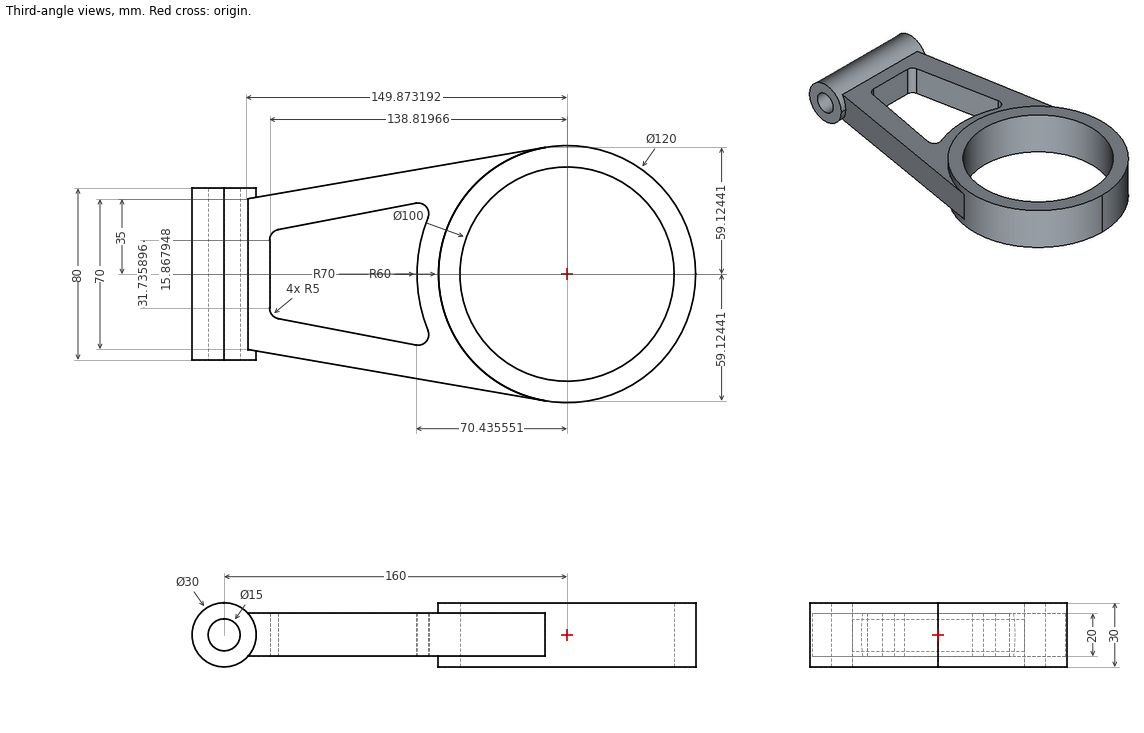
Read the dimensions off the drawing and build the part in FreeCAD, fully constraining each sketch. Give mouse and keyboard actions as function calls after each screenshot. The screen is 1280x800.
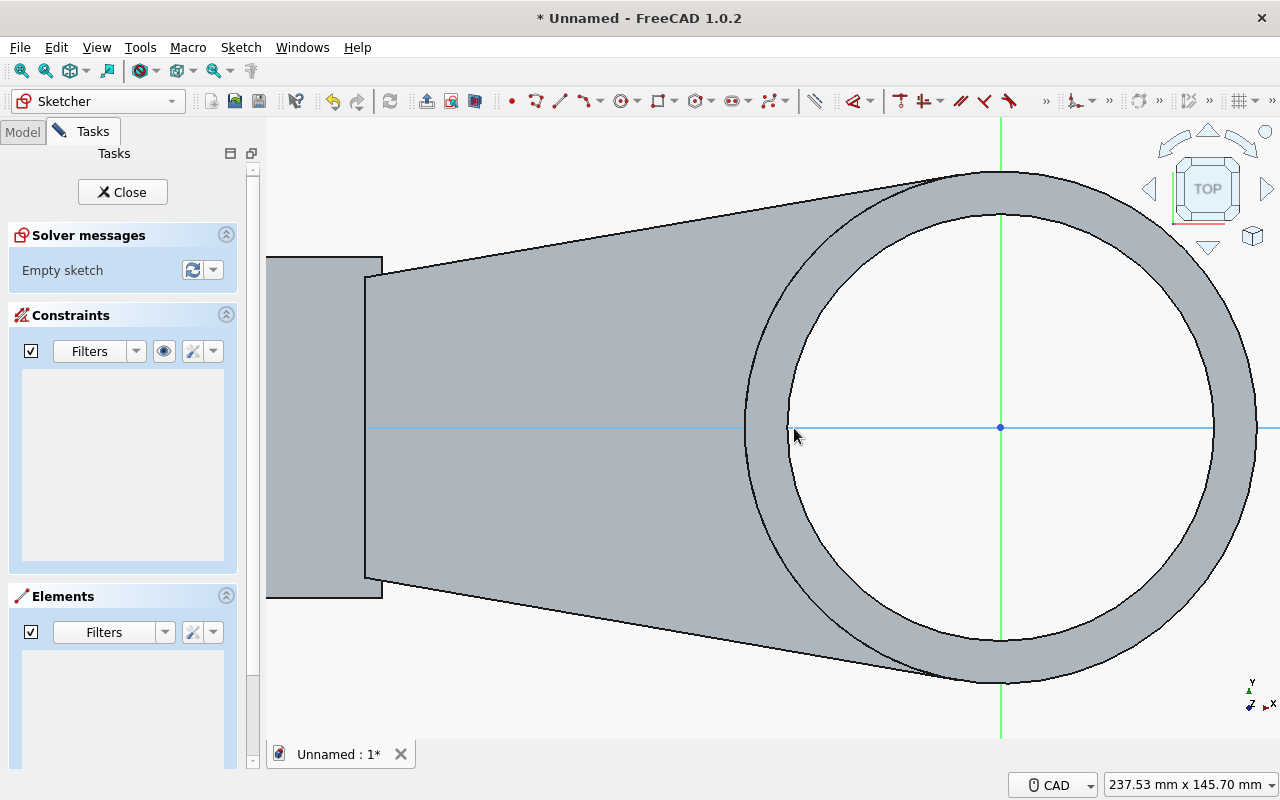
click(560, 102)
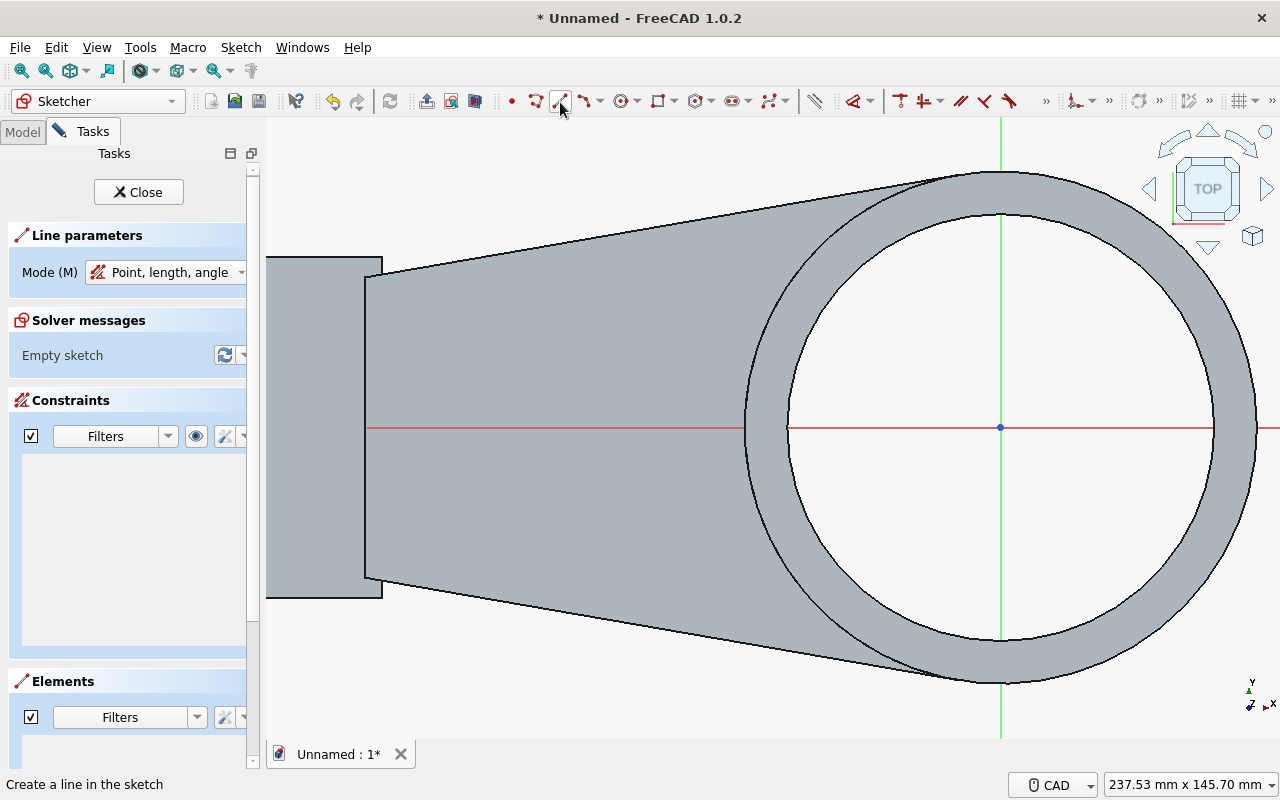
click(408, 360)
click(408, 495)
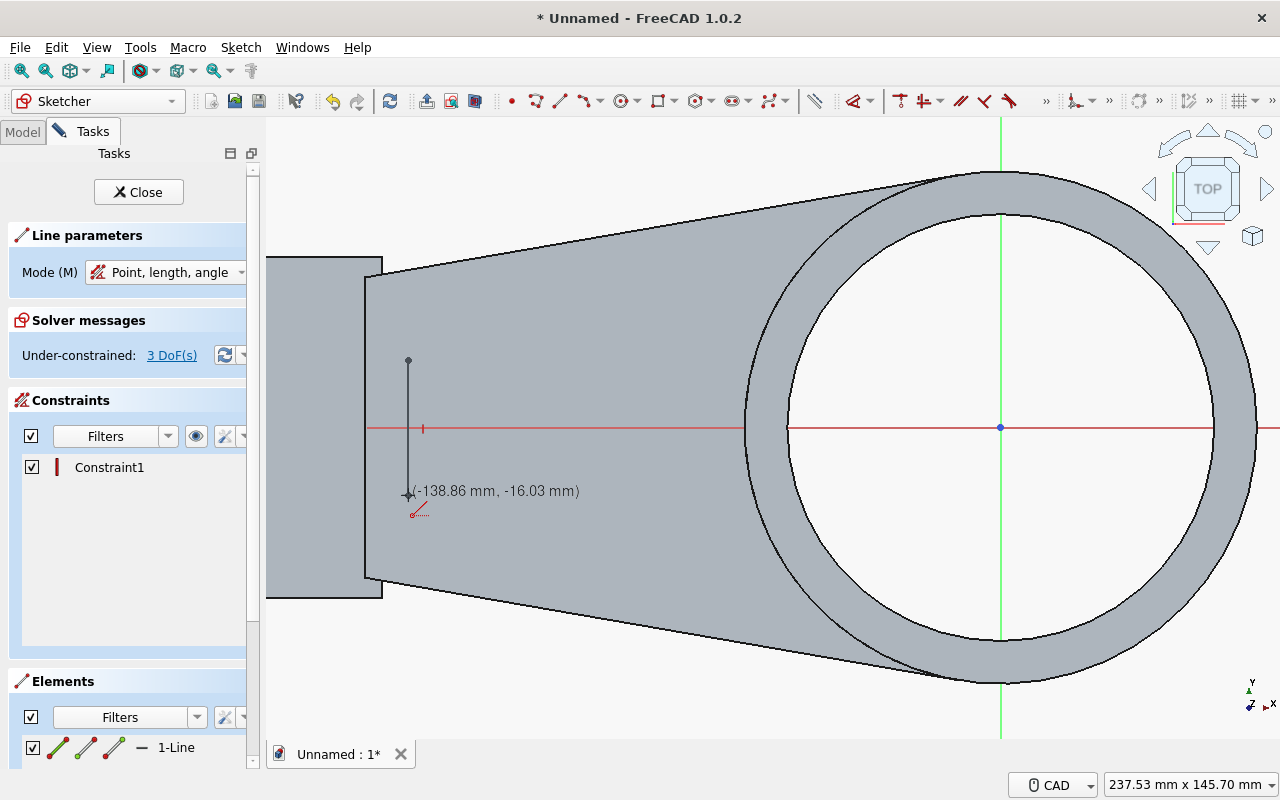
click(425, 516)
click(700, 569)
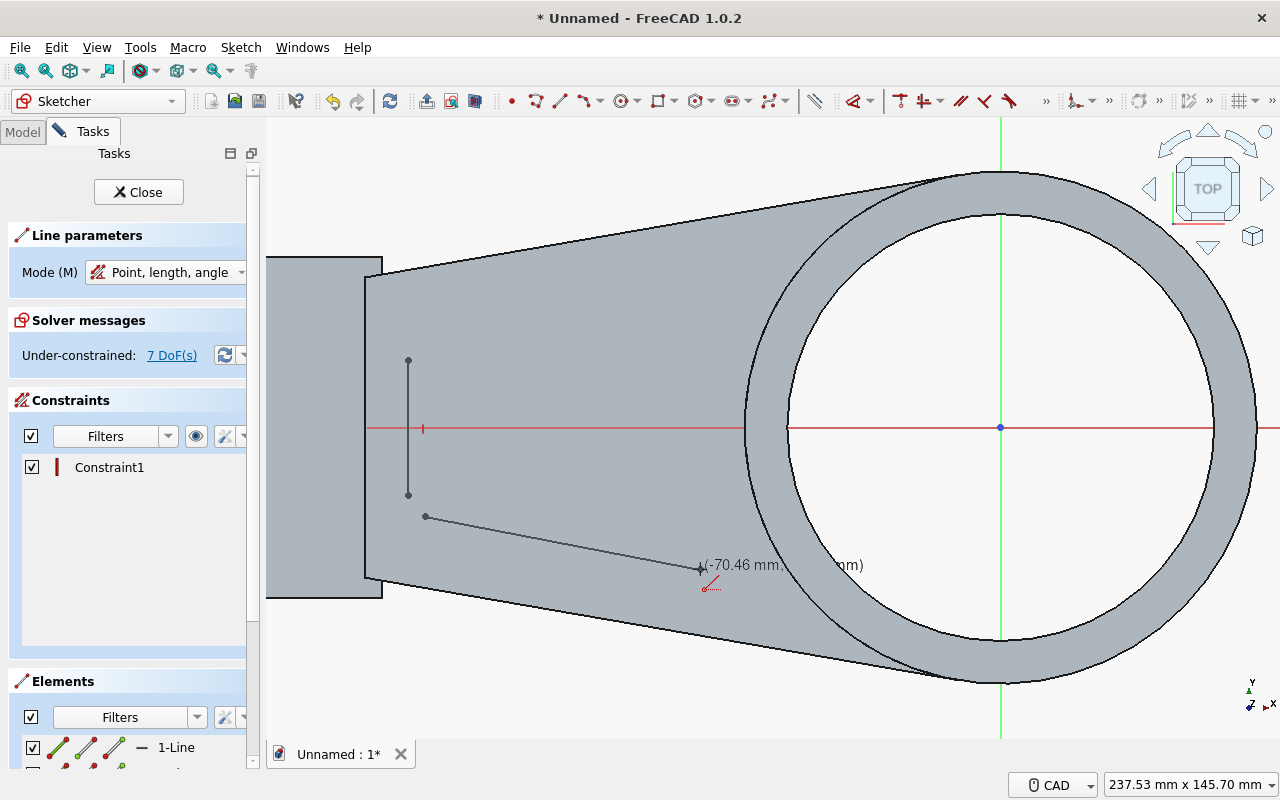
click(700, 286)
click(425, 339)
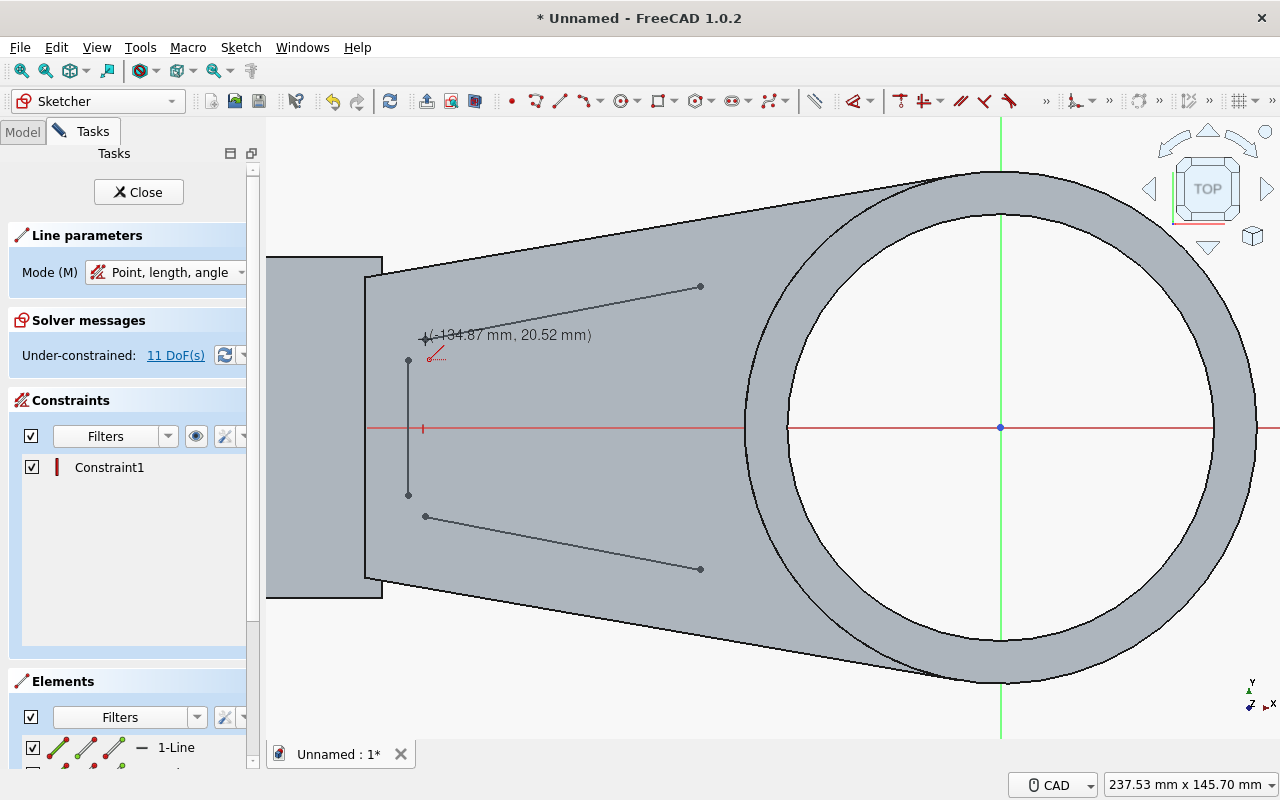
click(584, 102)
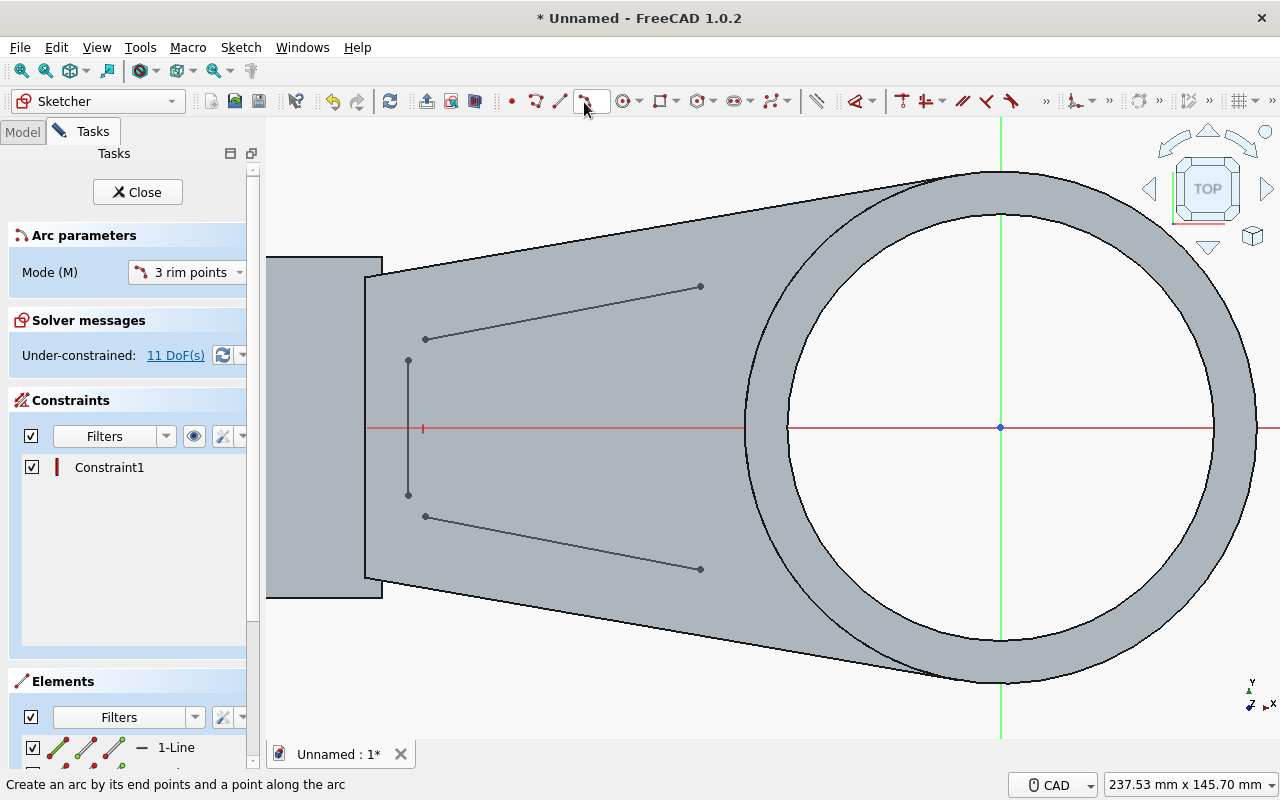
click(408, 496)
click(425, 517)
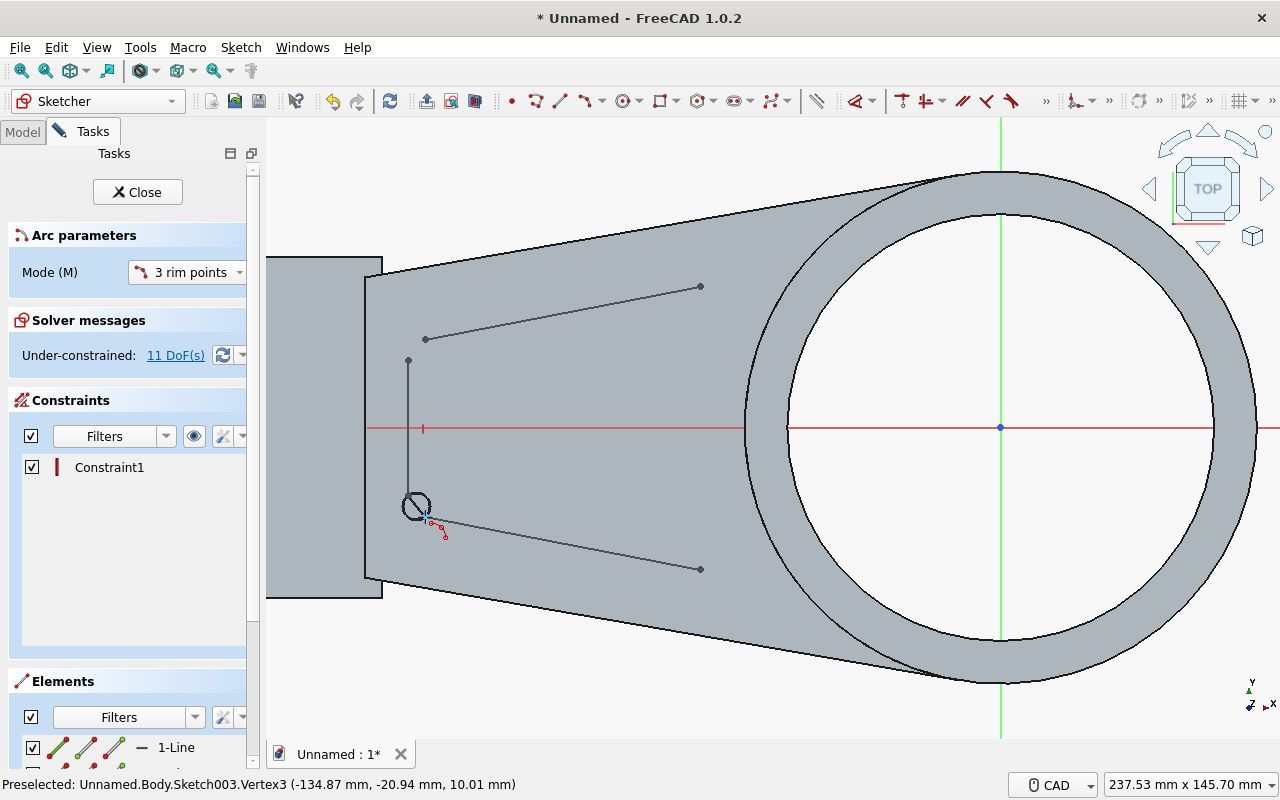
scroll(413, 509, up, 6)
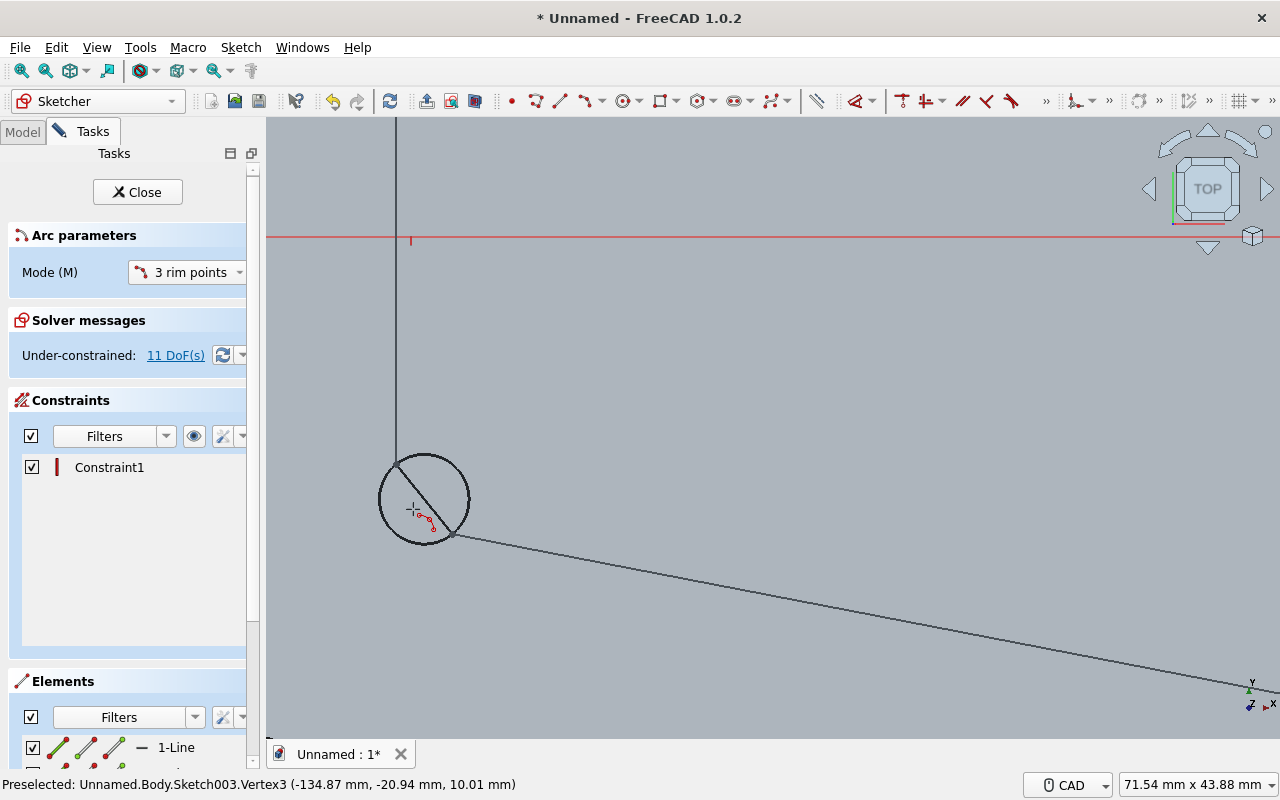
click(413, 507)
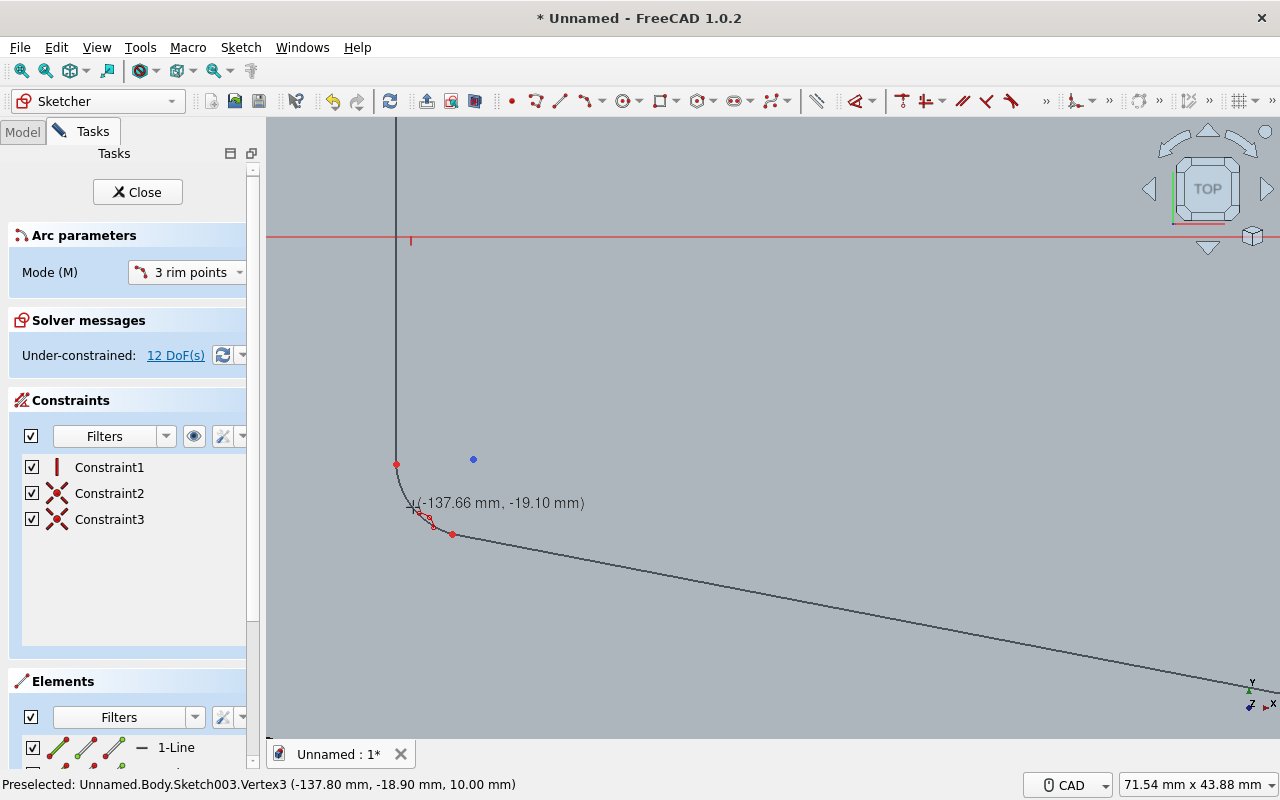
scroll(413, 510, down, 6)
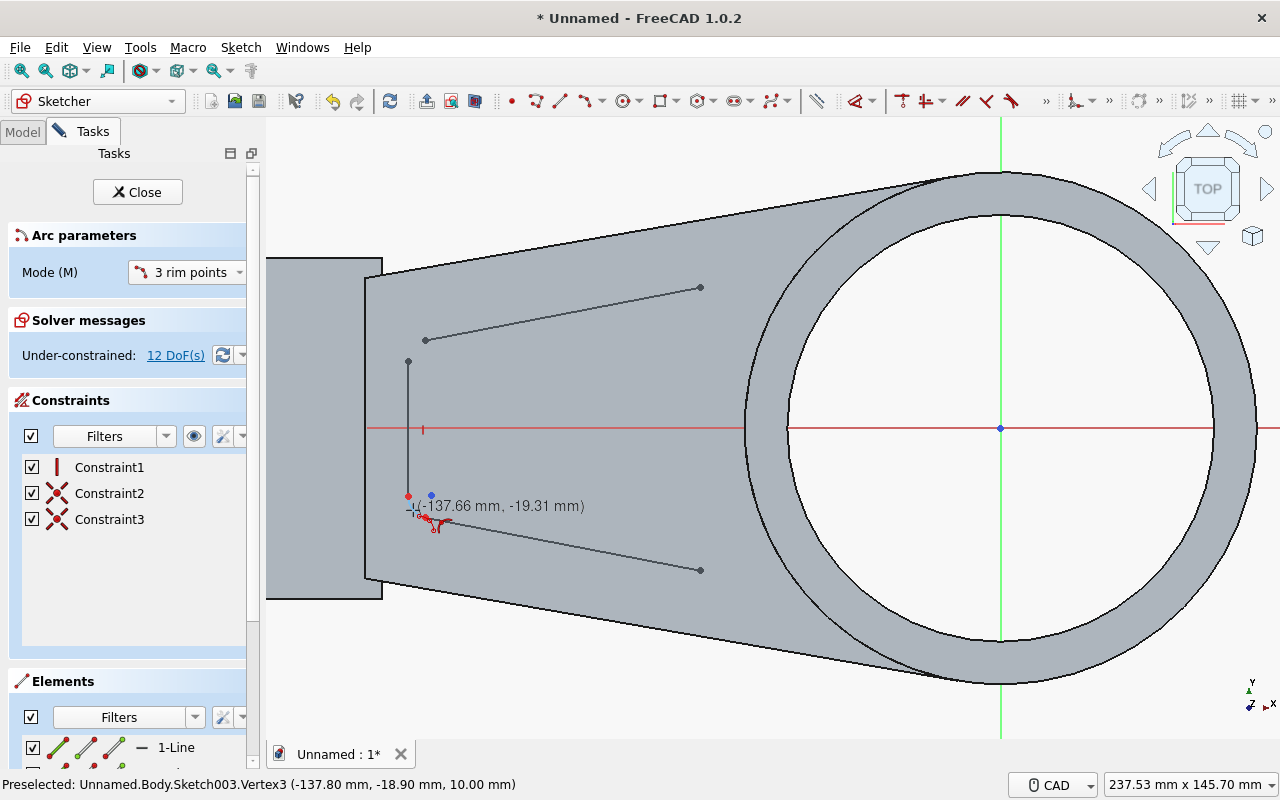
click(700, 571)
click(724, 541)